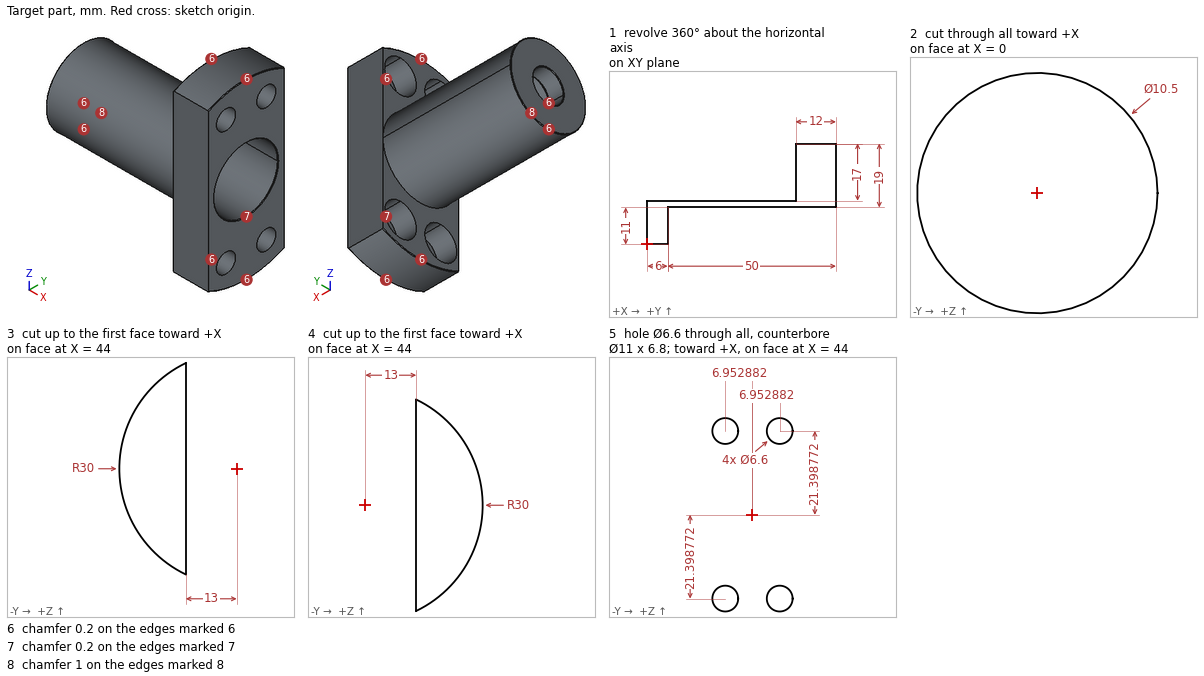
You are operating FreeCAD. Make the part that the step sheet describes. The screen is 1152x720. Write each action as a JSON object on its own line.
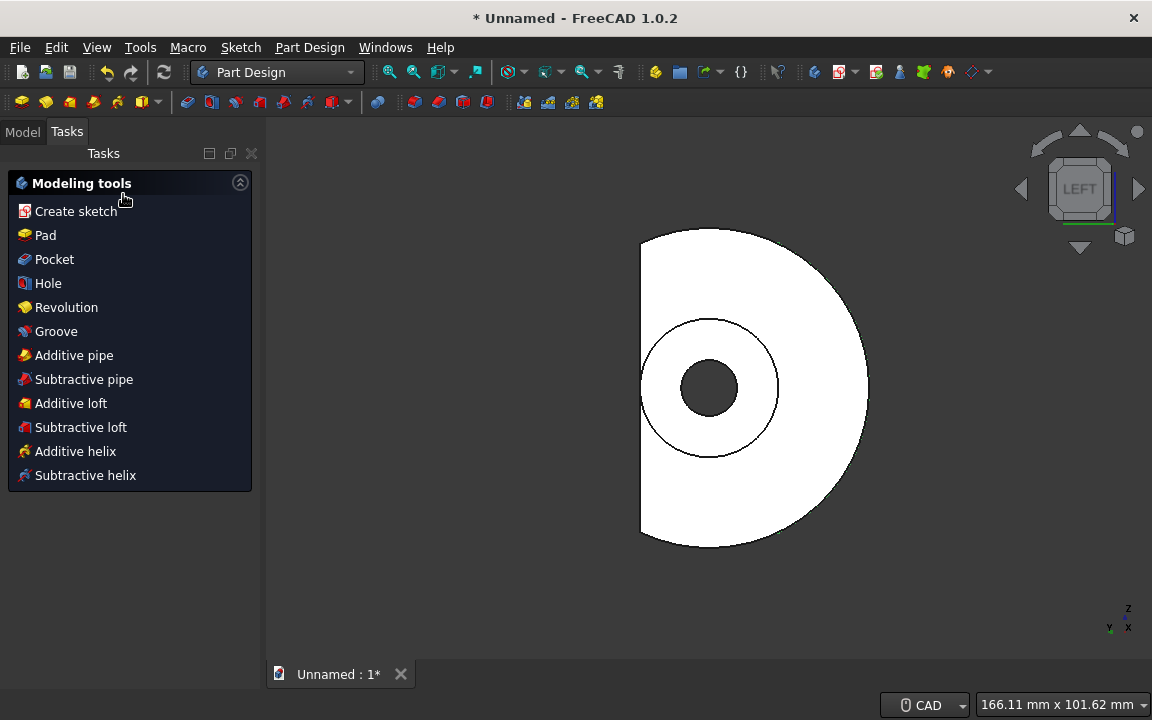
{"action": "left_click", "coordinate": [188, 102]}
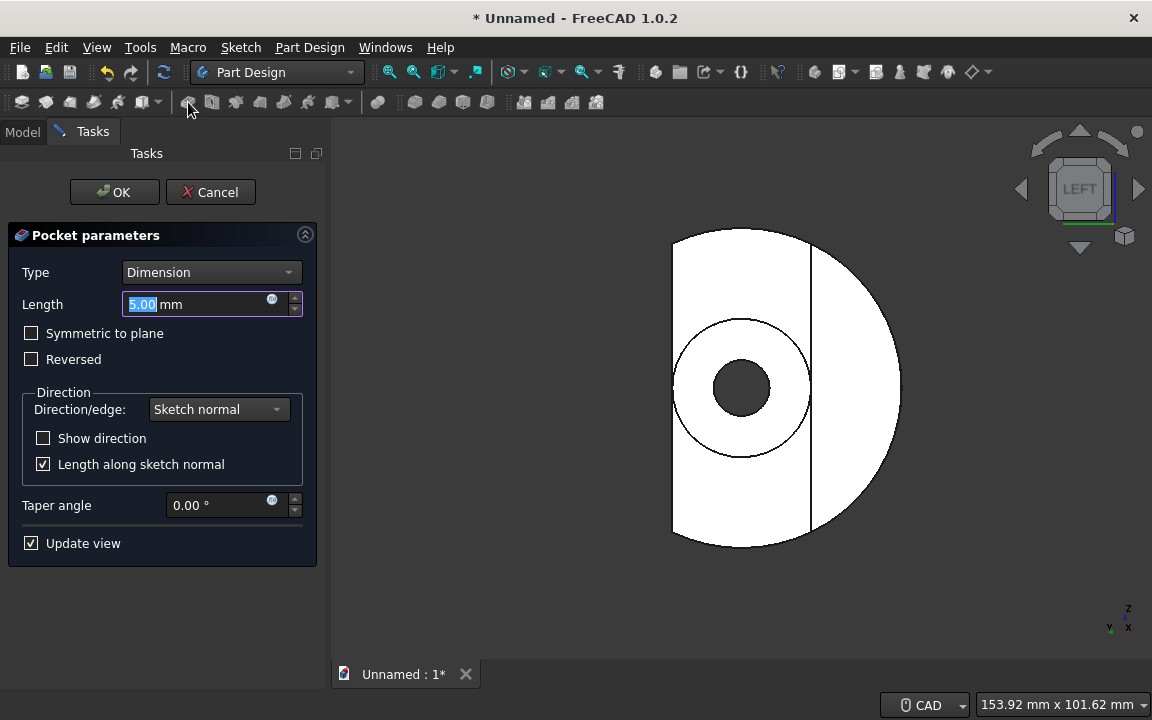
{"action": "left_click", "coordinate": [212, 272]}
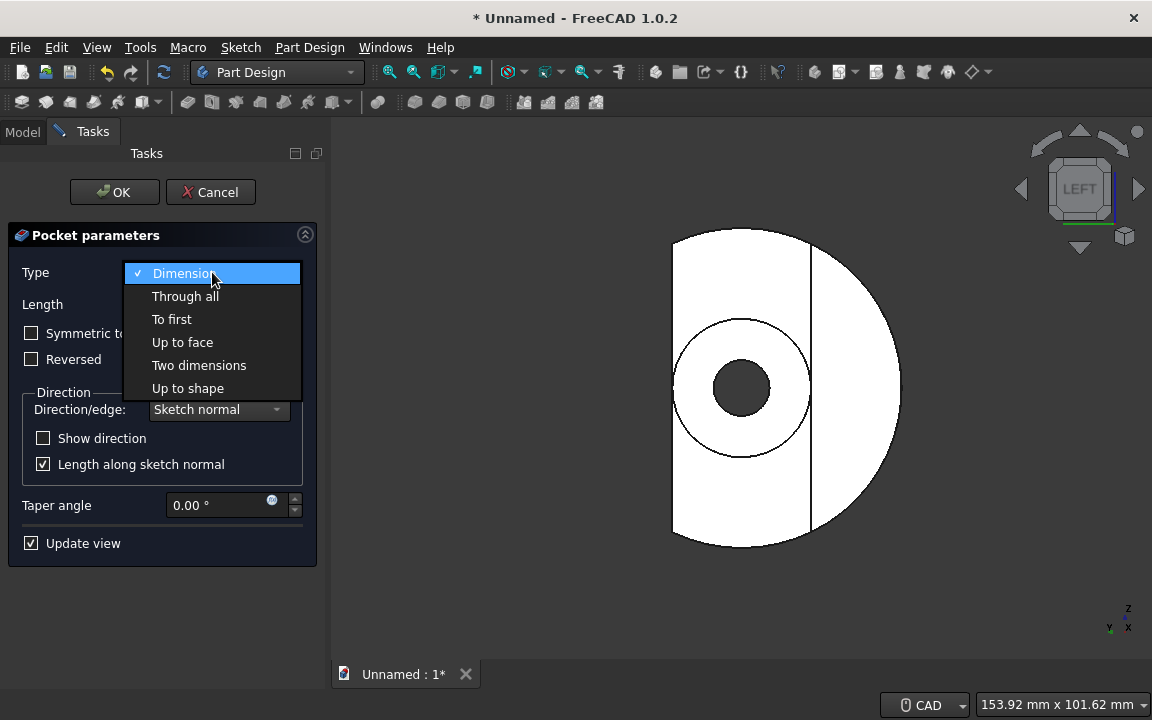
{"action": "left_click", "coordinate": [212, 320]}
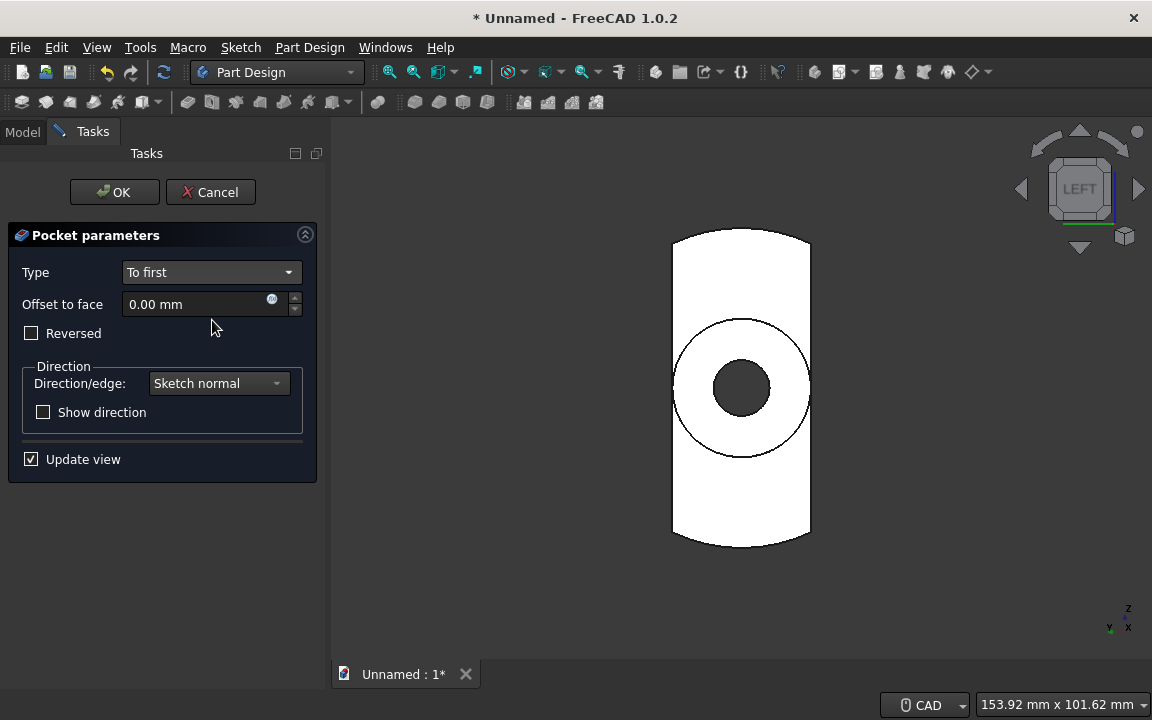
{"action": "left_click", "coordinate": [115, 192]}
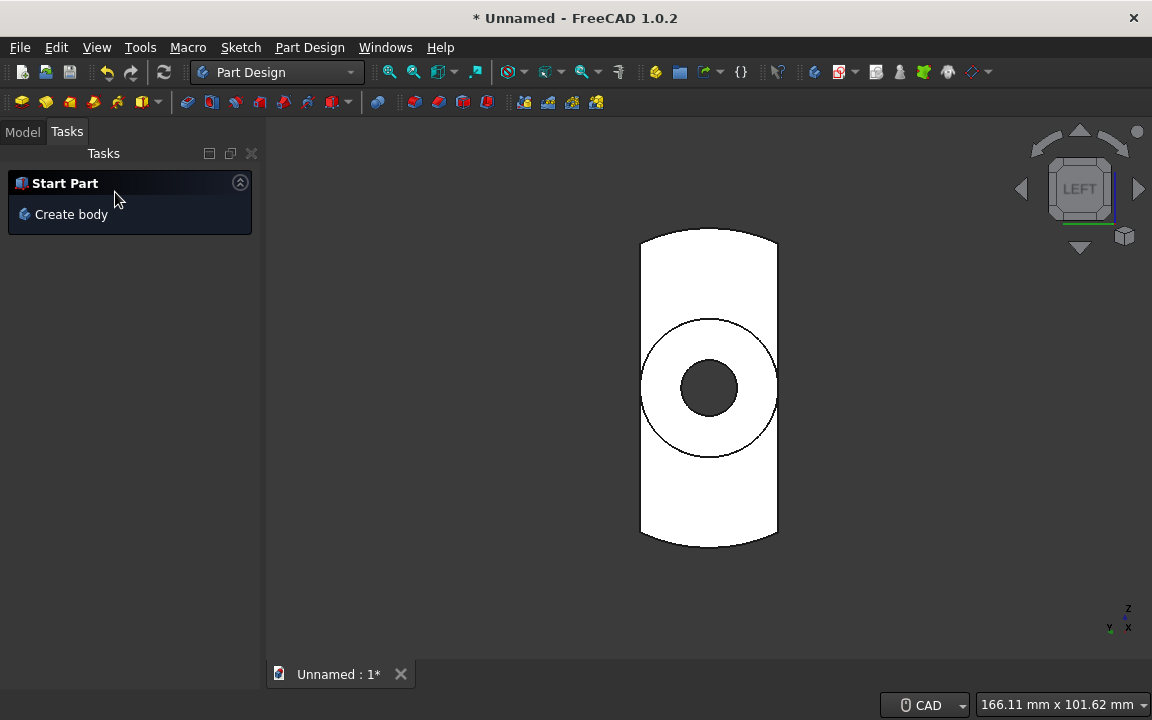
{"action": "left_click", "coordinate": [689, 490]}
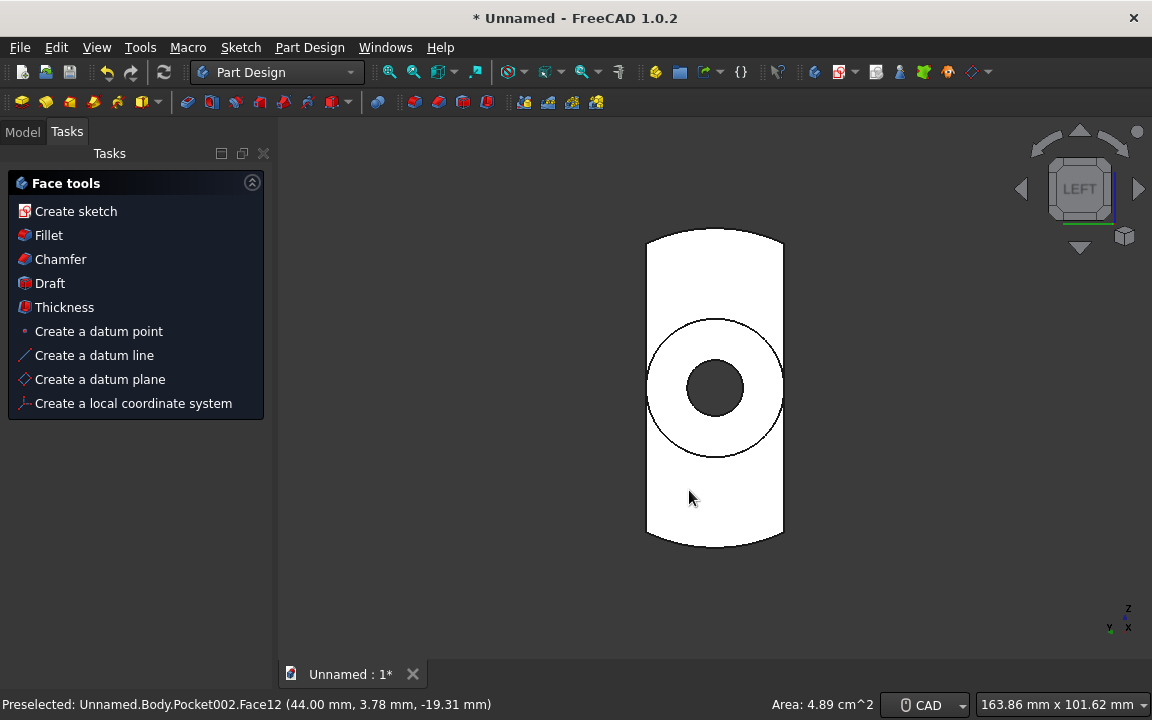
{"action": "left_click", "coordinate": [840, 72]}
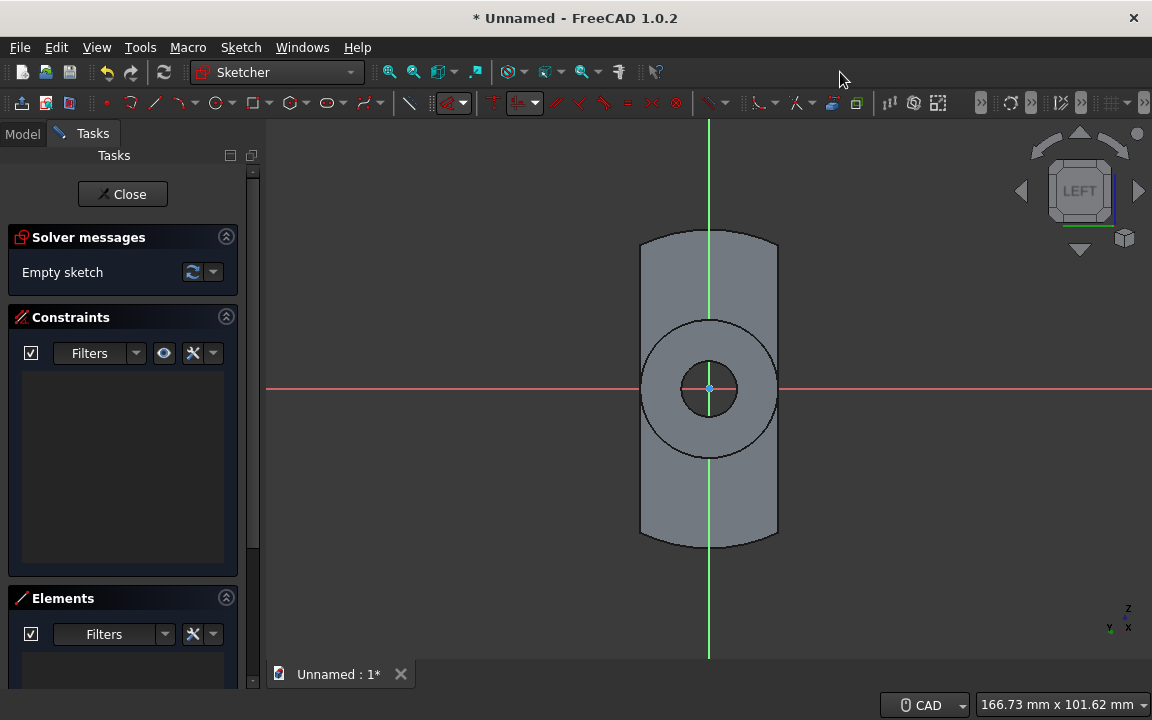
{"action": "left_click", "coordinate": [70, 104]}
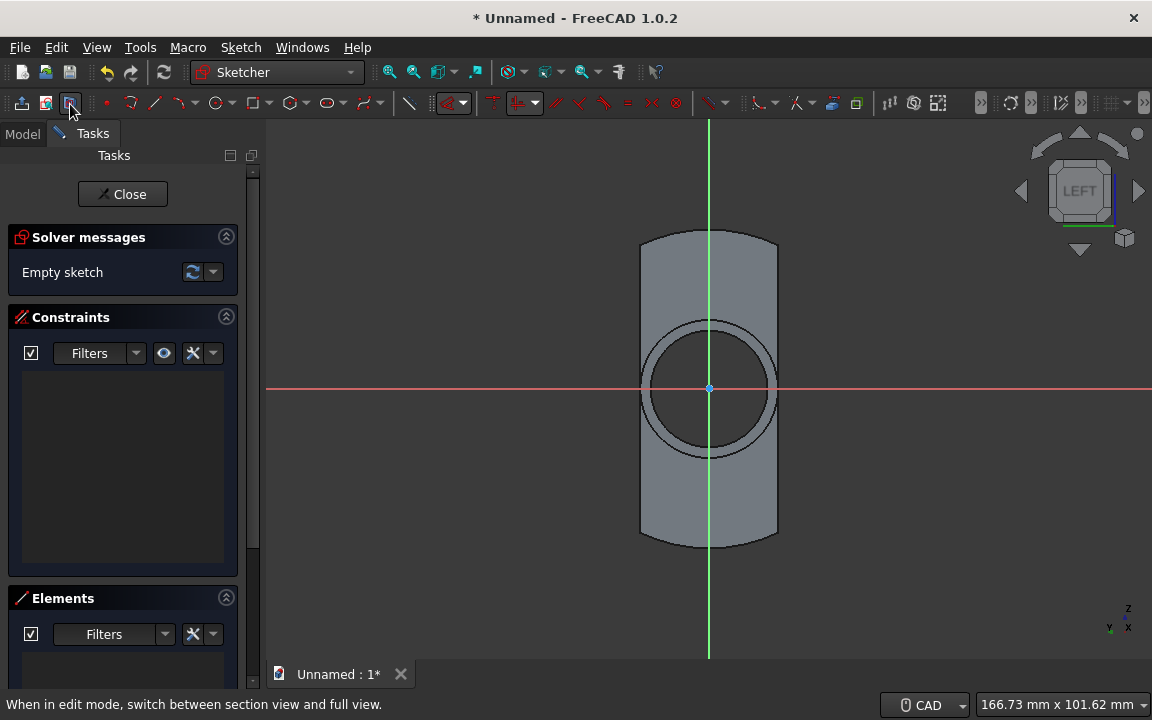
{"action": "key", "text": "g c"}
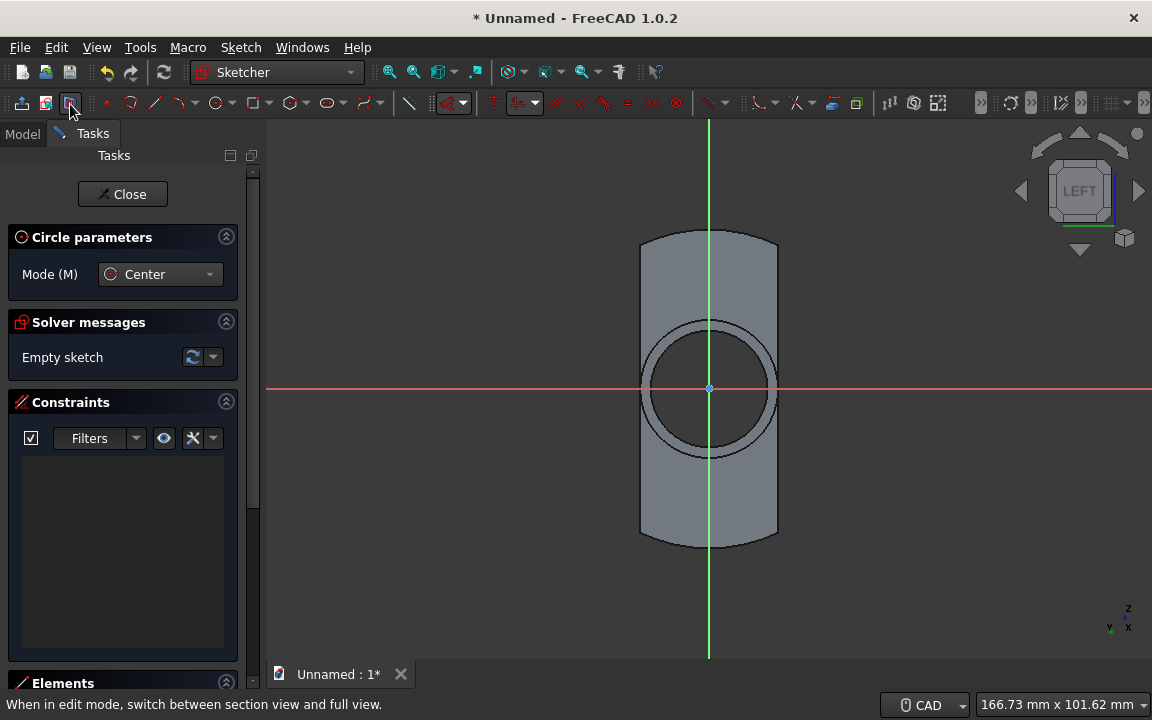
{"action": "scroll", "coordinate": [746, 275], "scroll_direction": "up", "scroll_amount": 2}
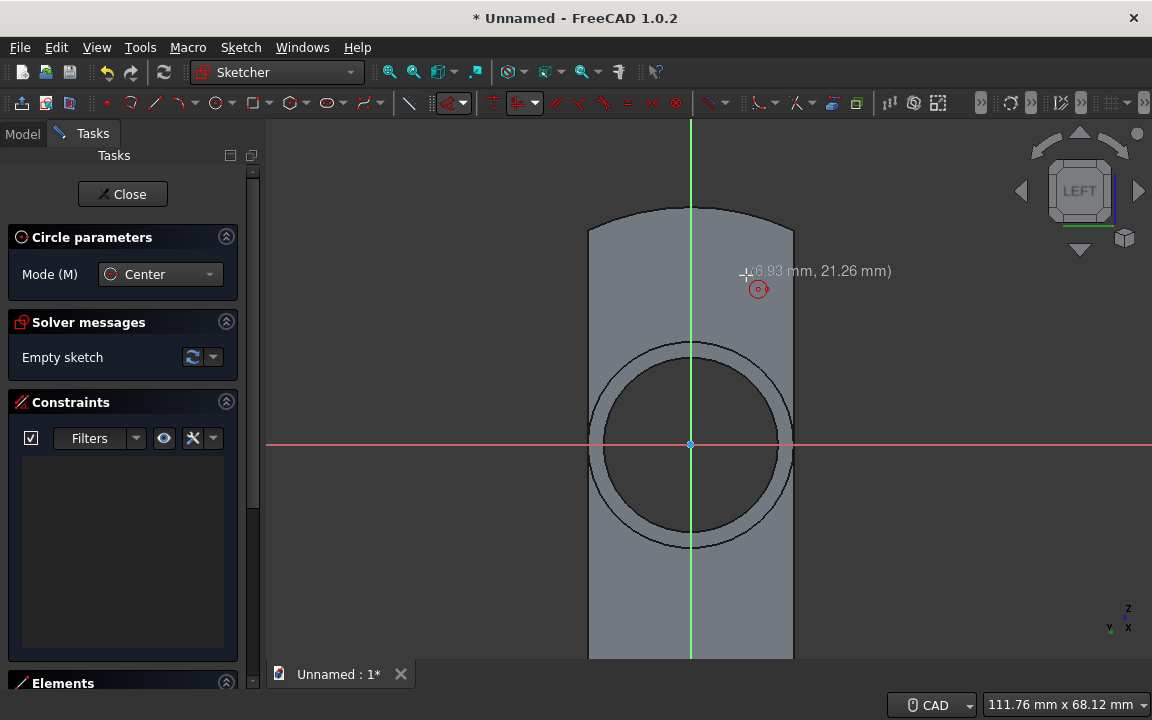
{"action": "left_click", "coordinate": [746, 275]}
{"action": "mouse_move", "coordinate": [764, 257]}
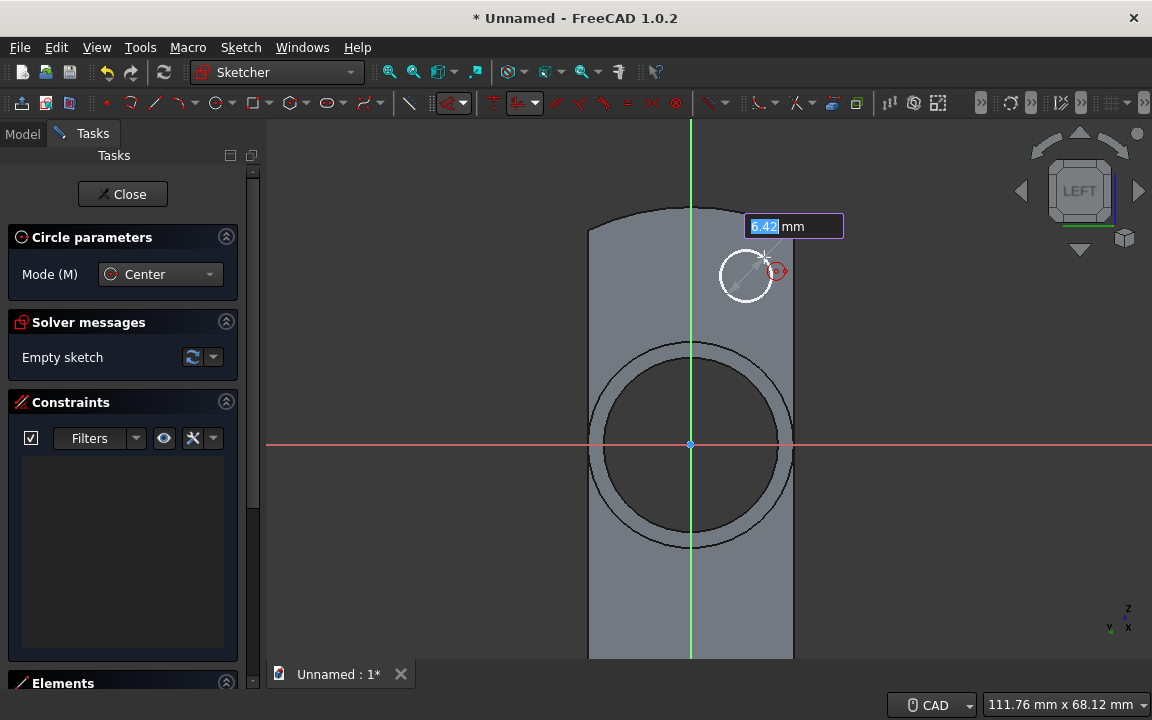
{"action": "type", "text": "6.6"}
{"action": "key", "text": "Return"}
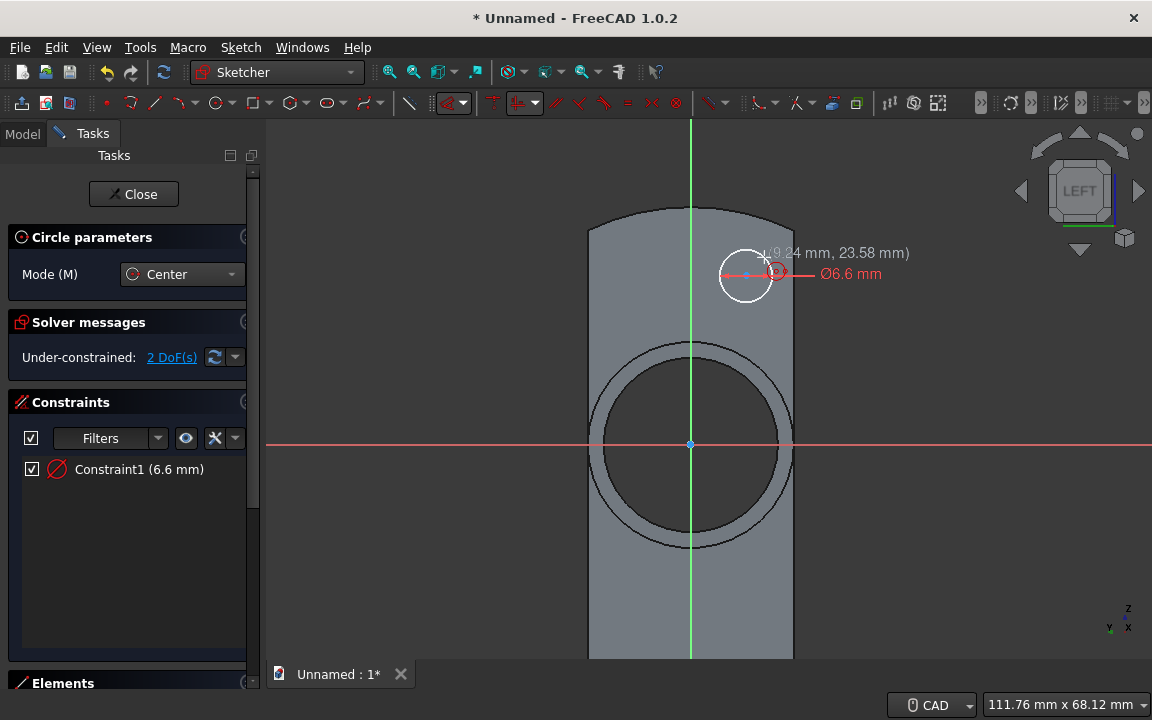
{"action": "left_click", "coordinate": [636, 275]}
{"action": "mouse_move", "coordinate": [654, 257]}